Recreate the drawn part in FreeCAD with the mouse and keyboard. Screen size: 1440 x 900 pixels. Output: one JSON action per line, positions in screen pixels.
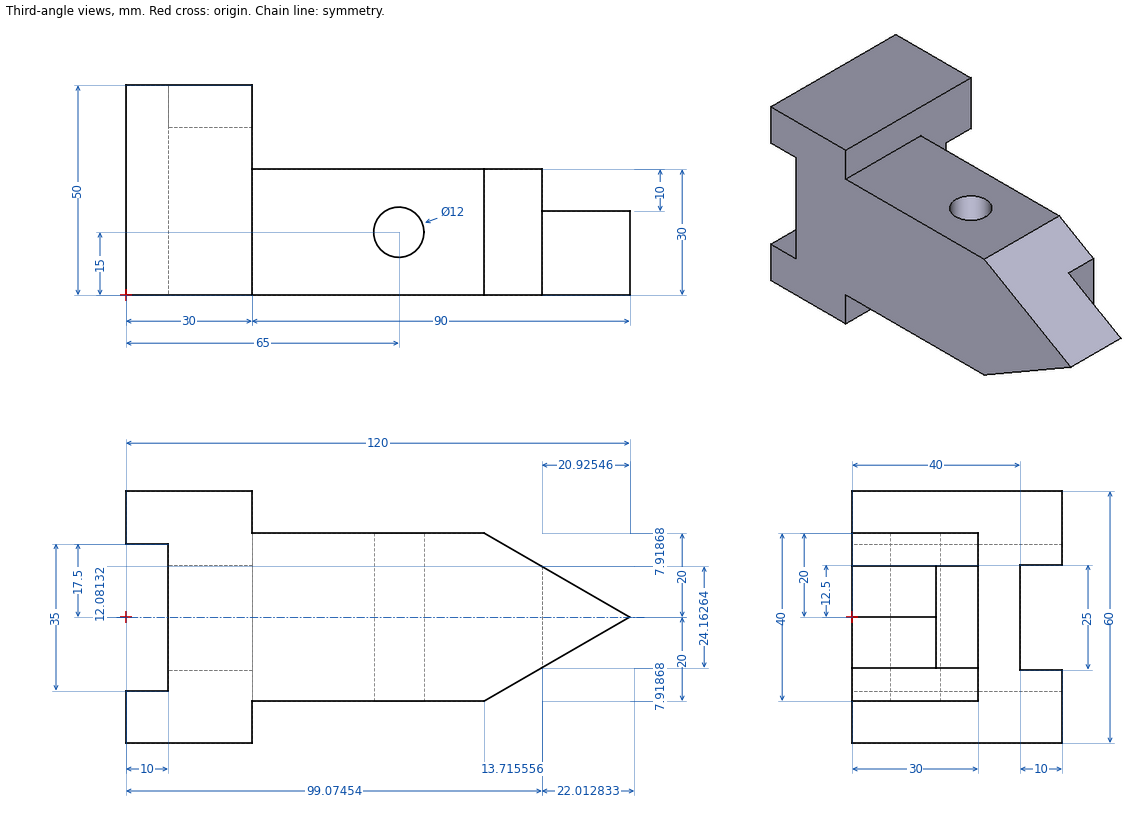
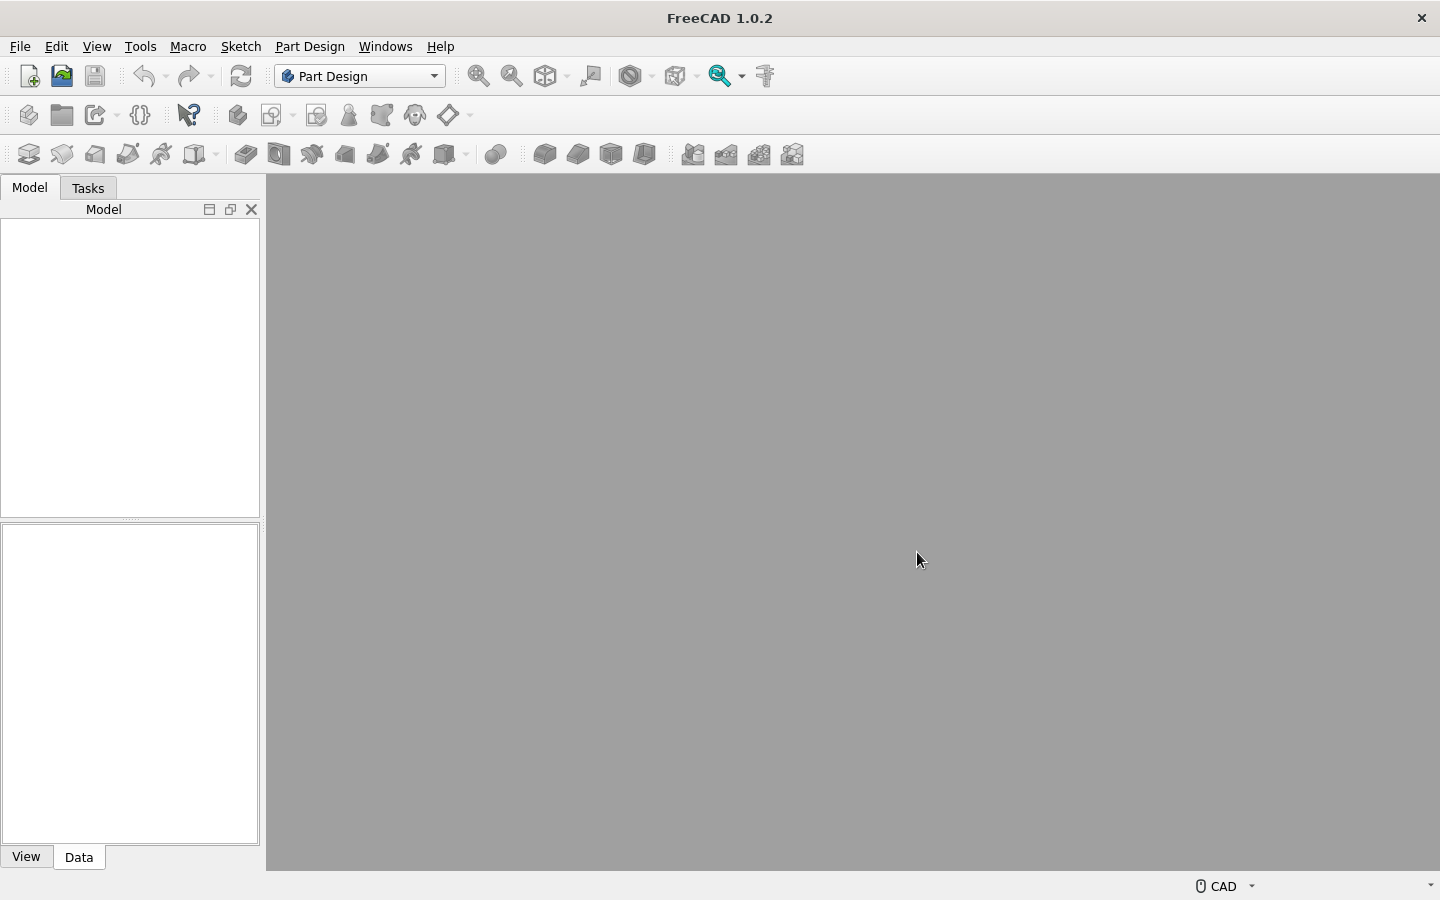
{"action": "left_click", "coordinate": [29, 76]}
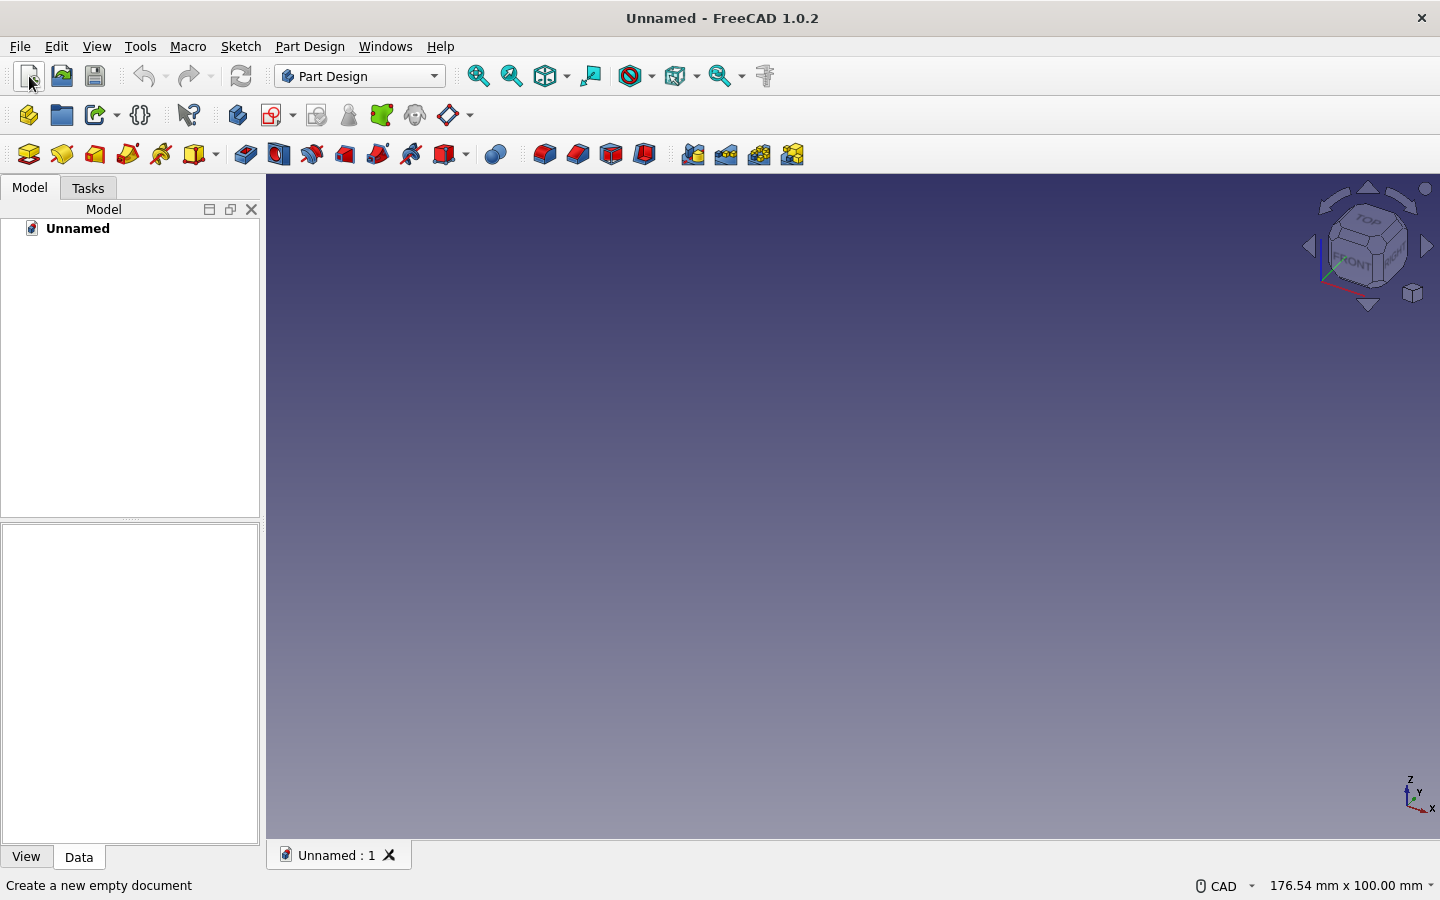
{"action": "left_click", "coordinate": [270, 116]}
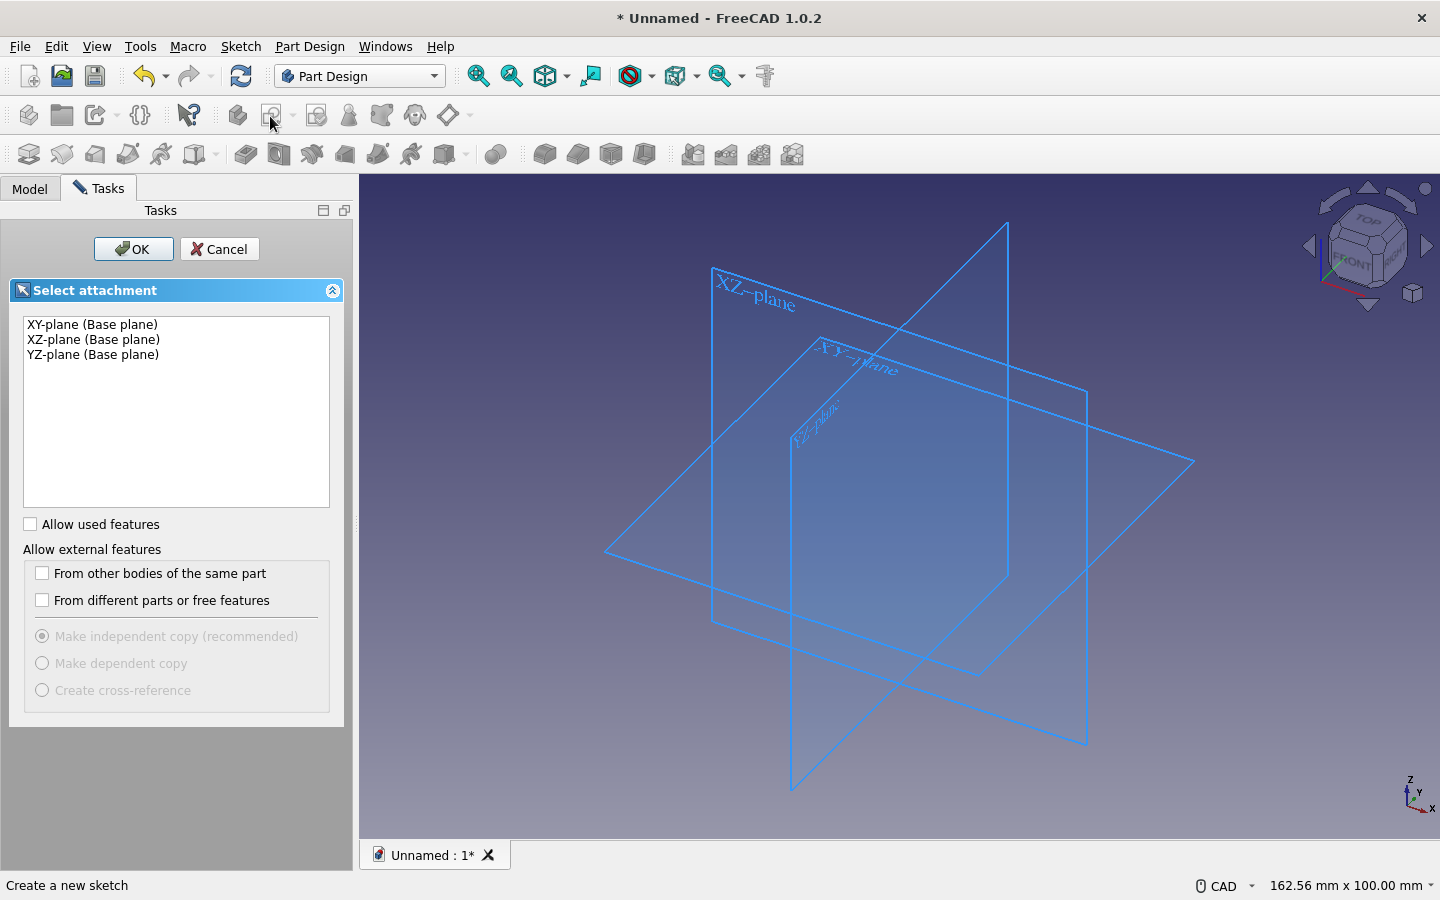
{"action": "left_click", "coordinate": [84, 324]}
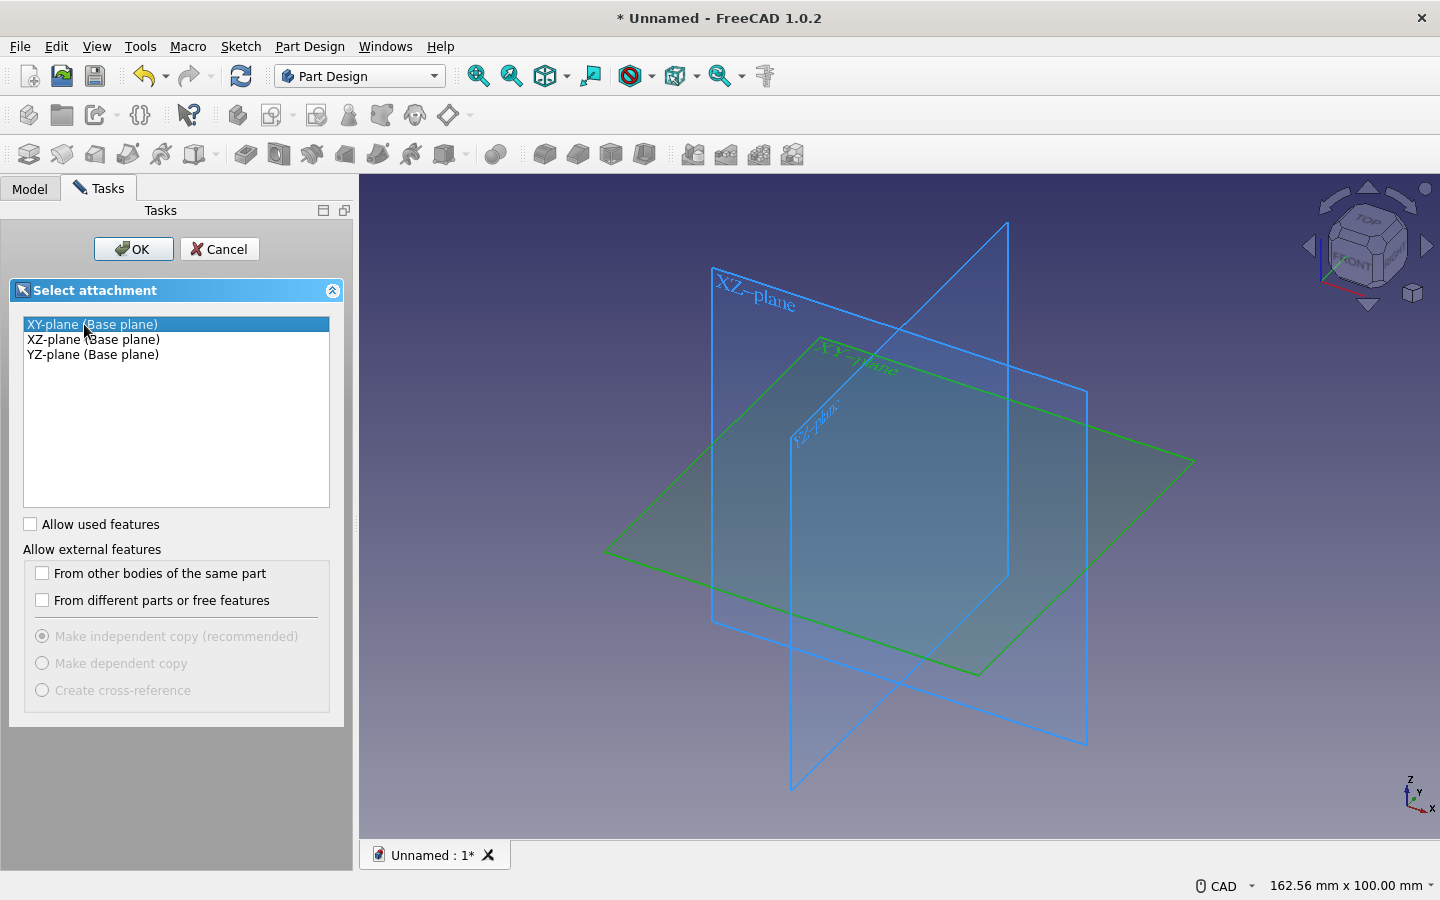
{"action": "left_click", "coordinate": [134, 249]}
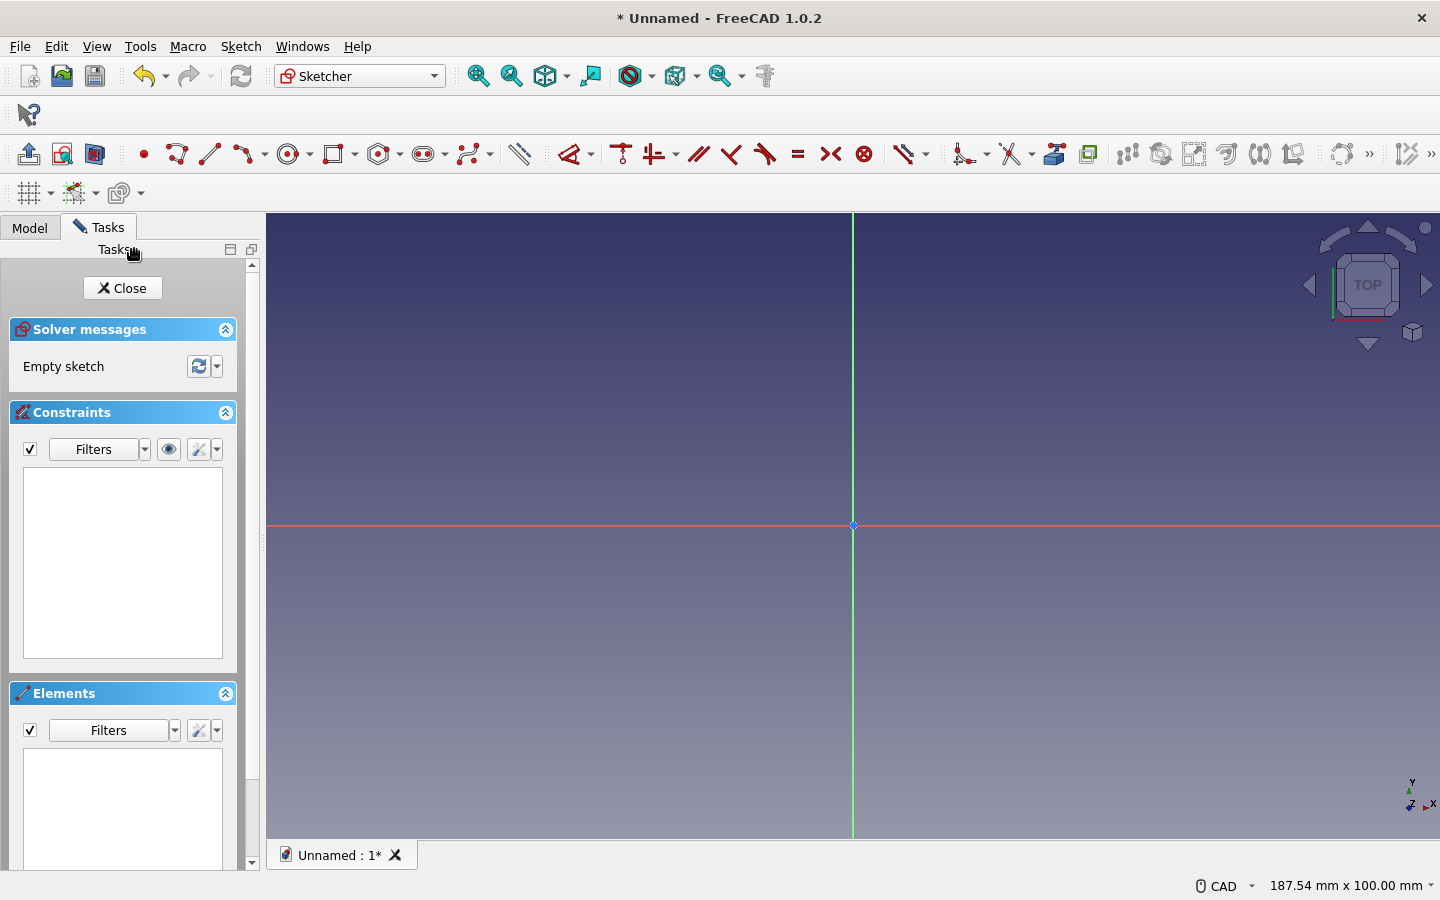
{"action": "scroll", "coordinate": [294, 811], "scroll_direction": "down", "scroll_amount": 1}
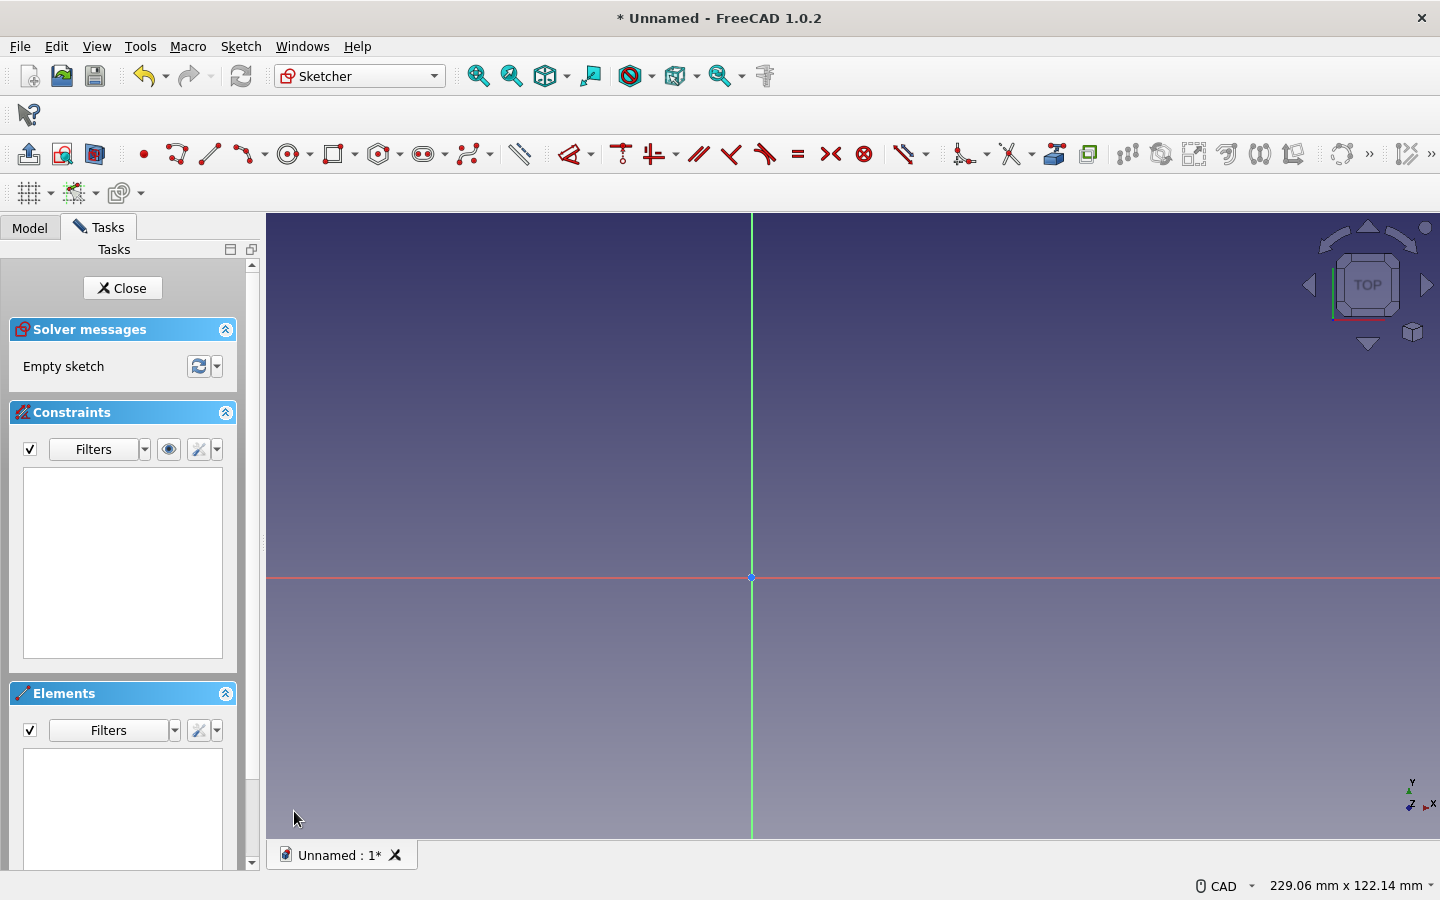
{"action": "scroll", "coordinate": [918, 295], "scroll_direction": "up", "scroll_amount": 2}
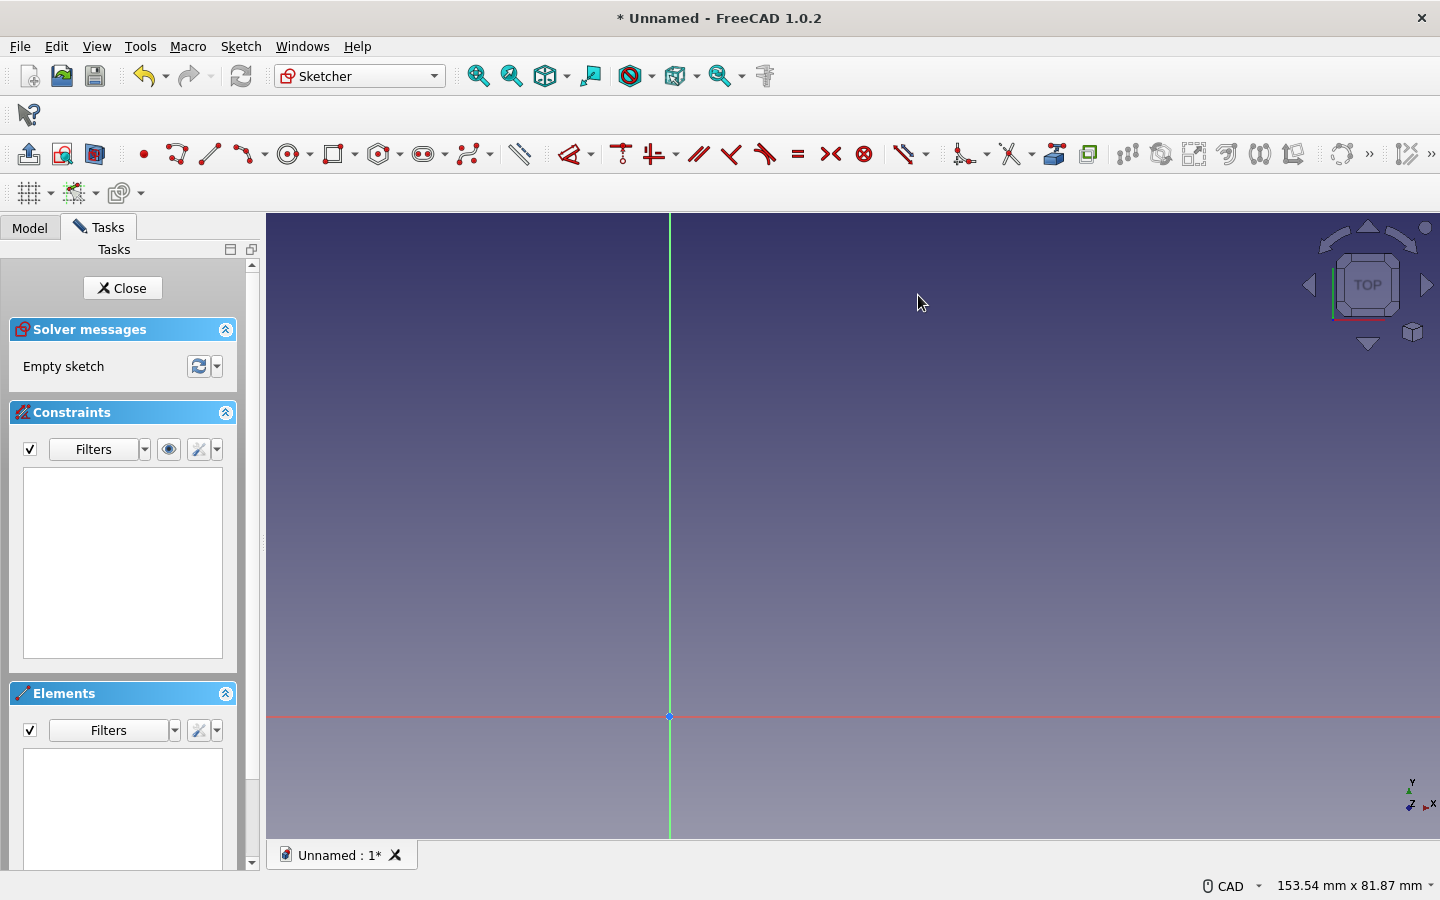
{"action": "left_click", "coordinate": [332, 154]}